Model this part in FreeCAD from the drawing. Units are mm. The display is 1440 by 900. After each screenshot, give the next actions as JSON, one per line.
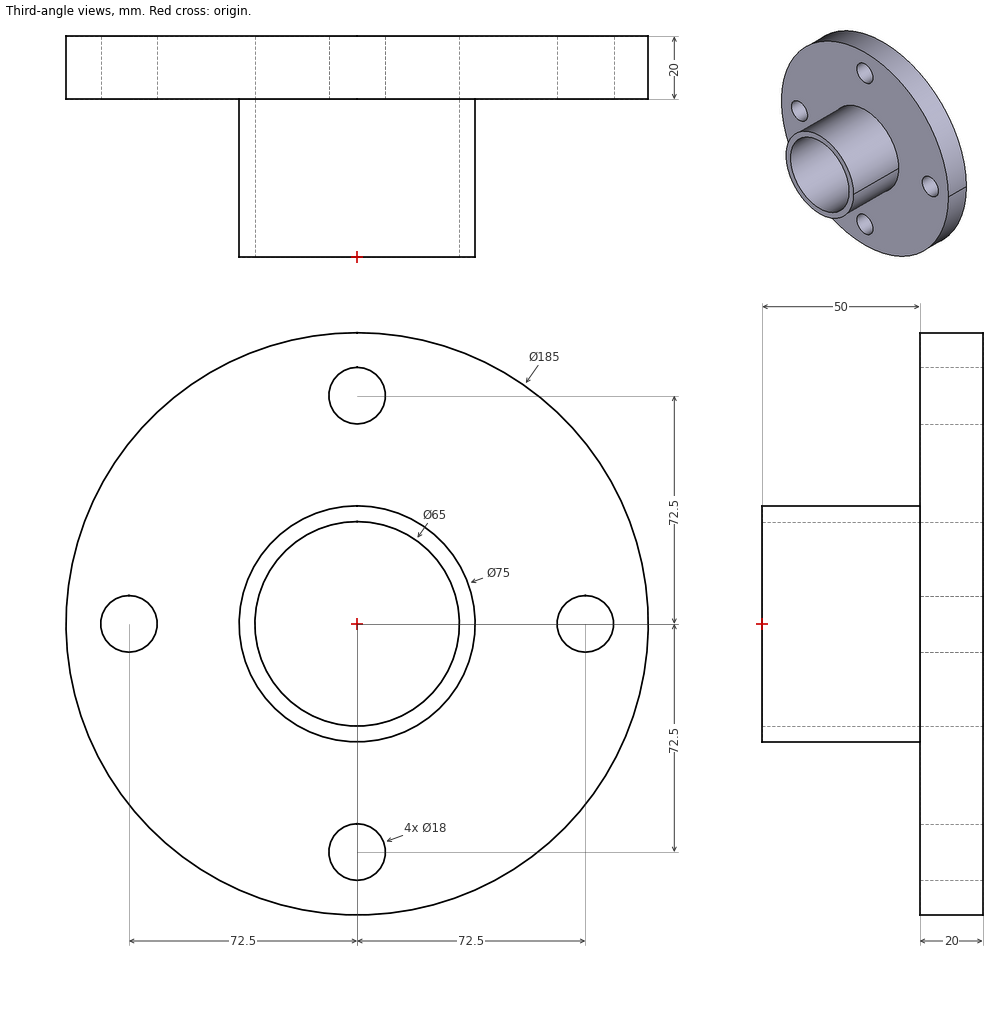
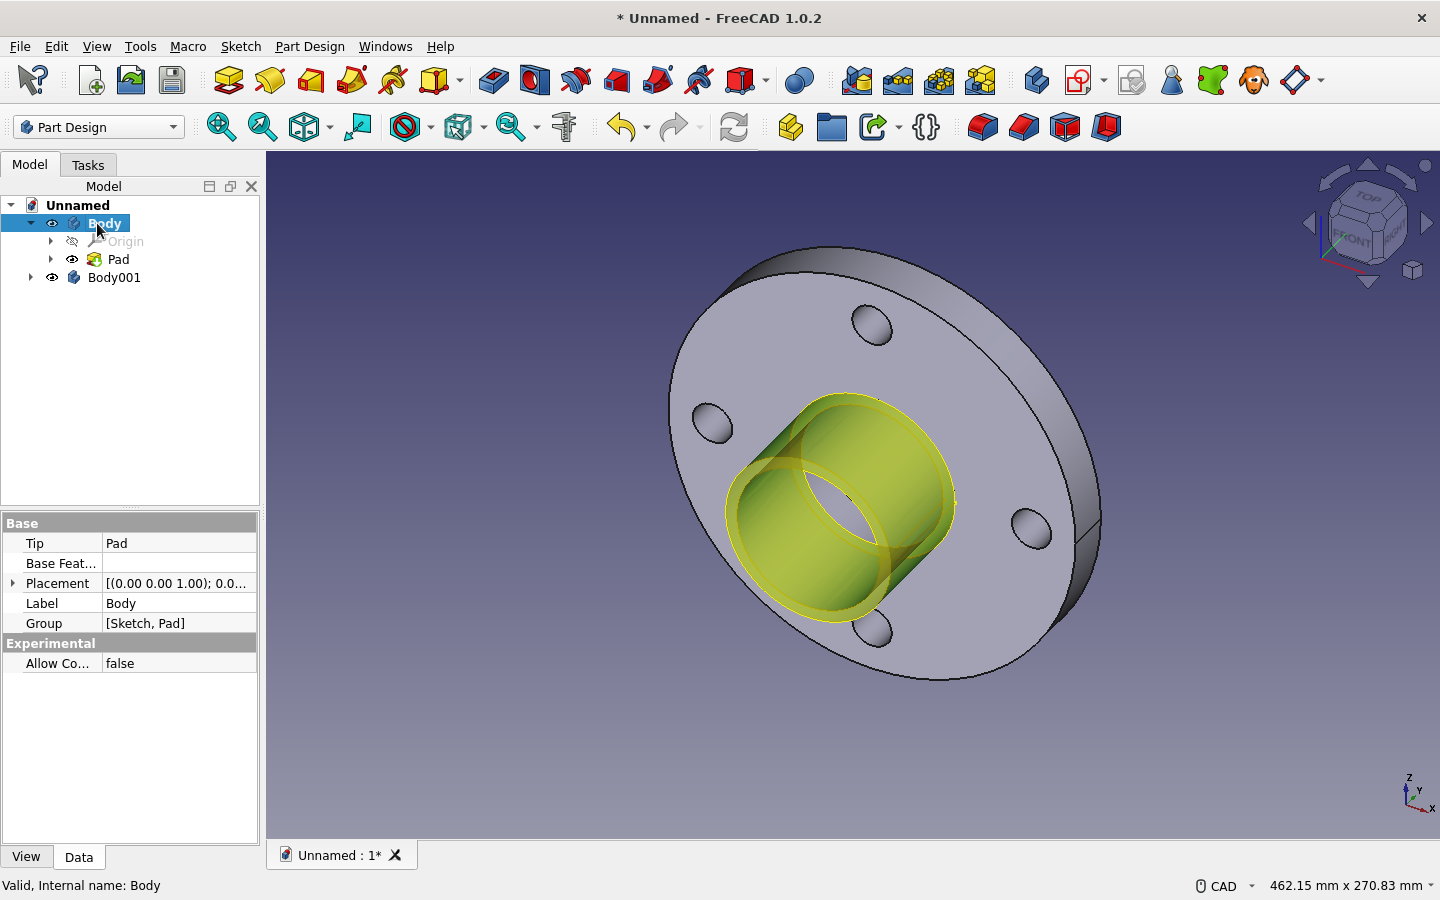
{"action": "left_click", "coordinate": [148, 663]}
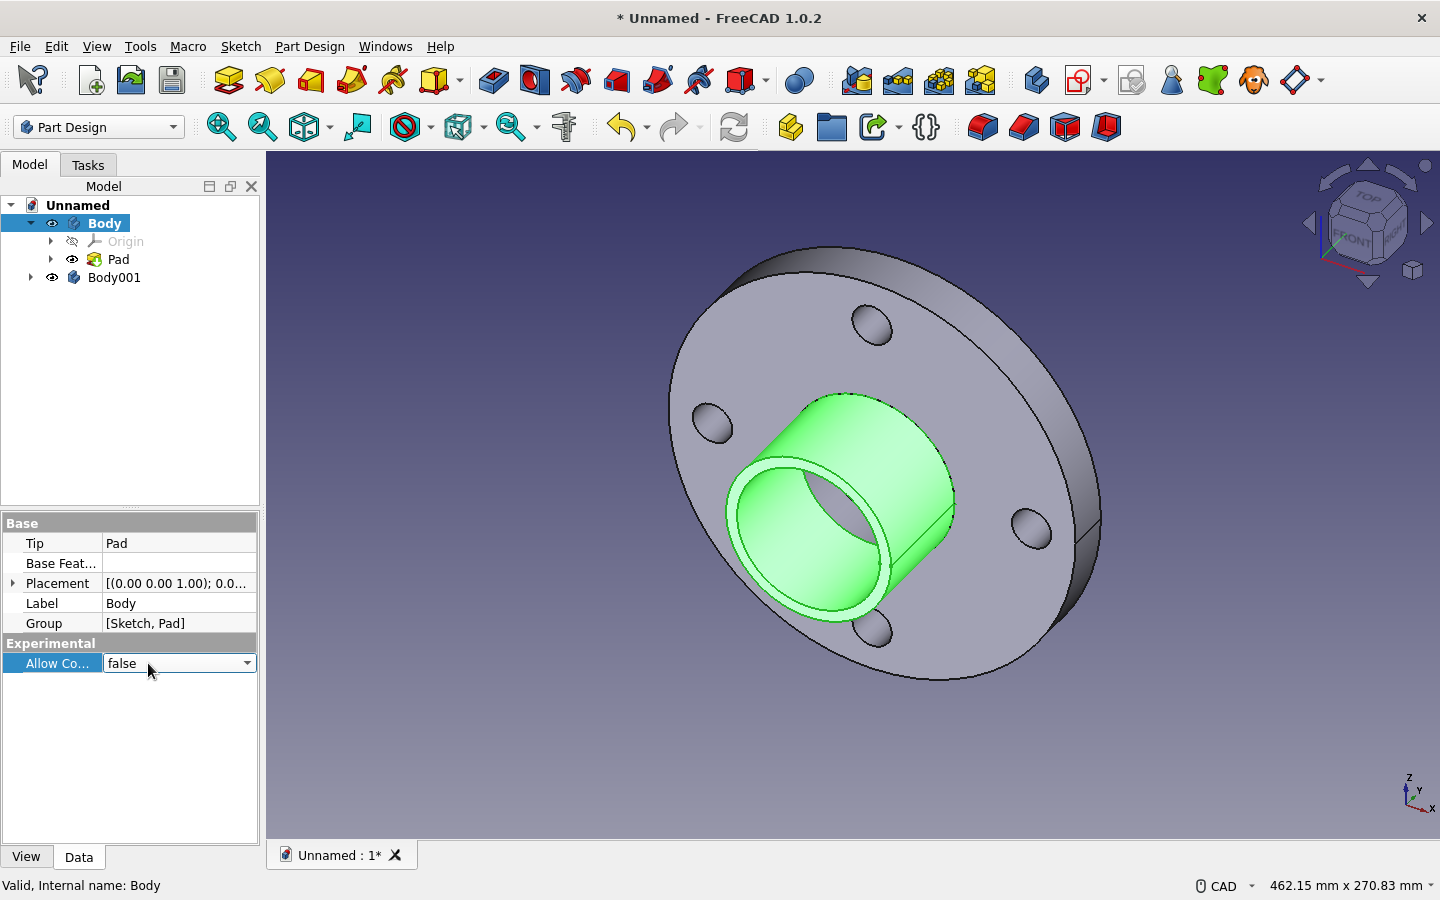
{"action": "left_click", "coordinate": [148, 663]}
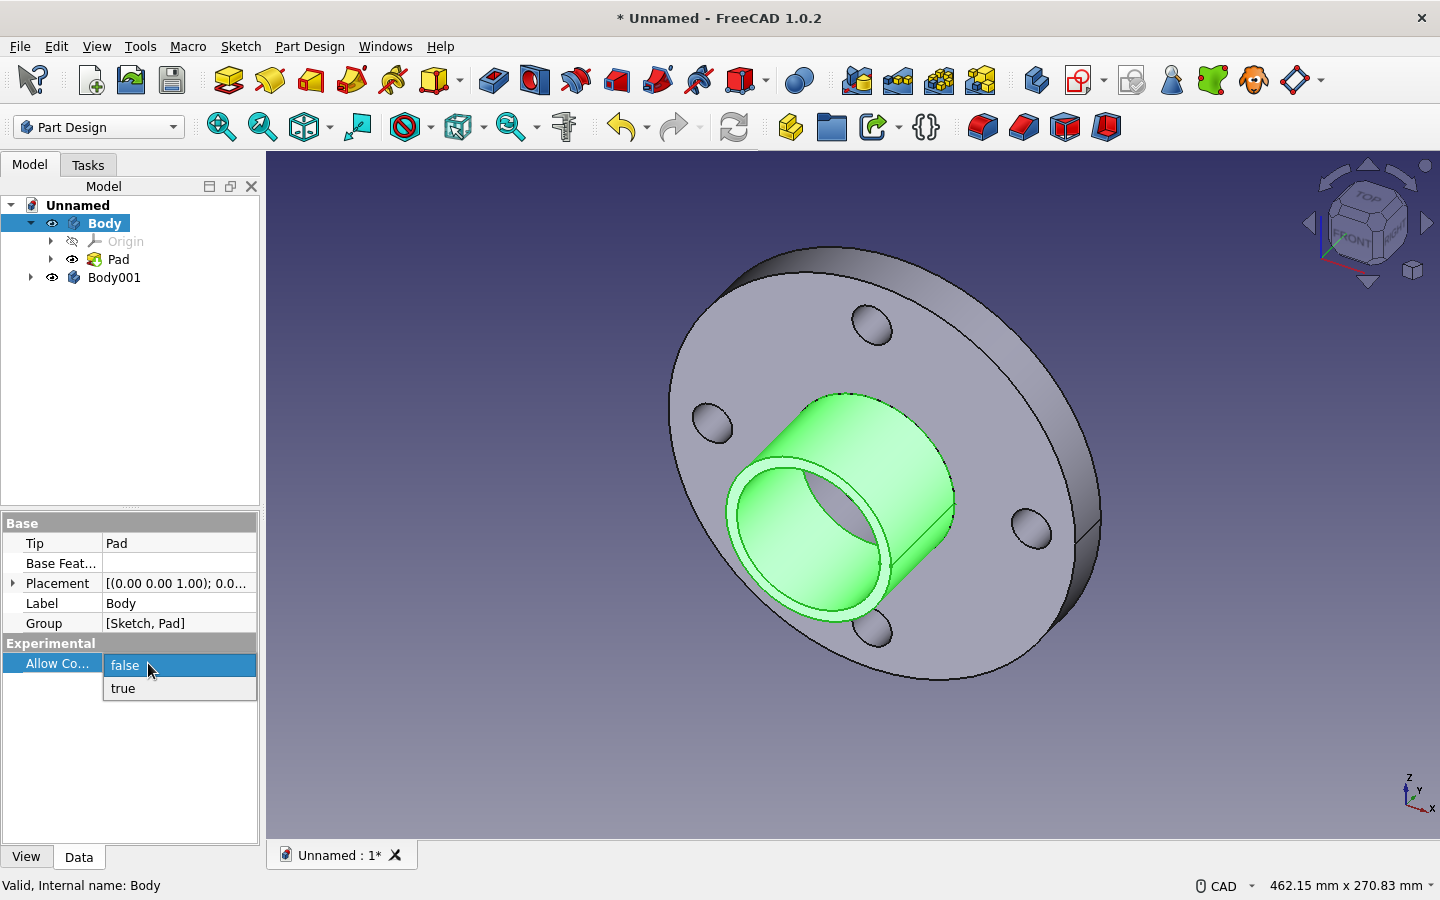
{"action": "left_click", "coordinate": [178, 688]}
{"action": "key", "text": "Return"}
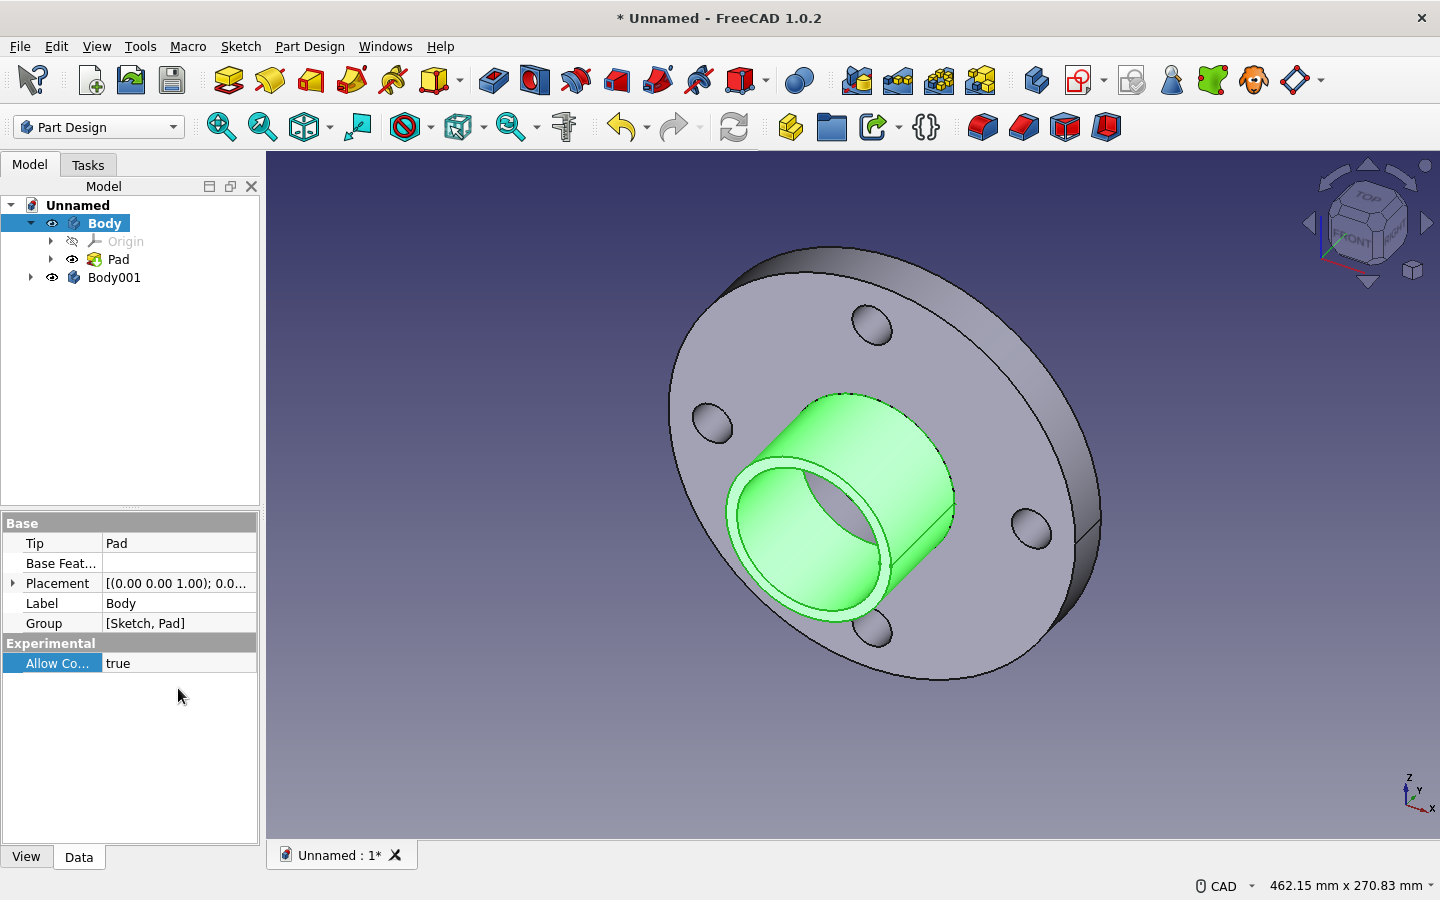
{"action": "left_click", "coordinate": [97, 277]}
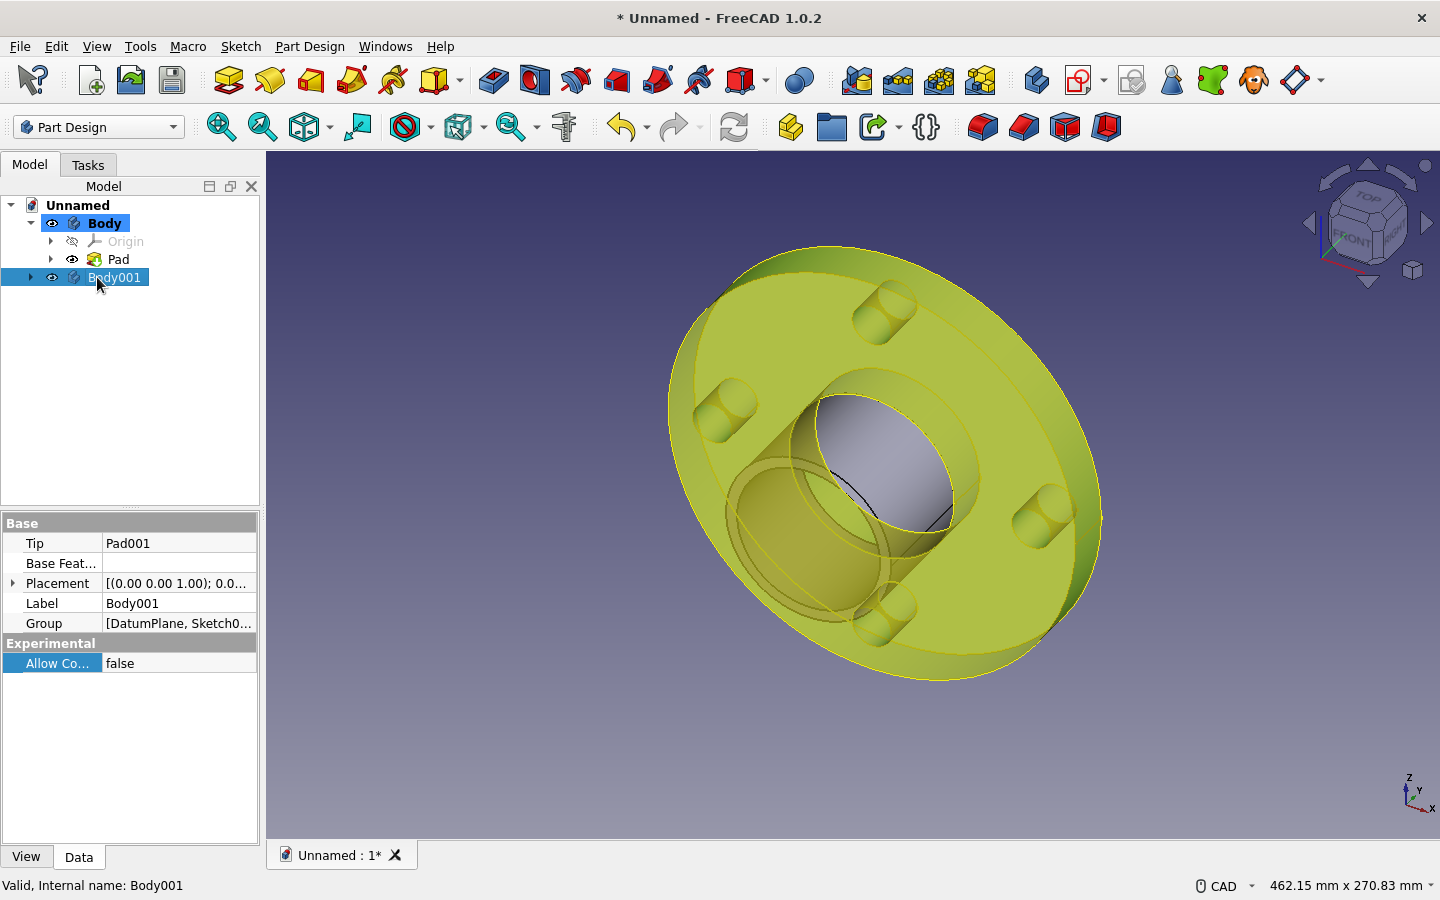
{"action": "left_click", "coordinate": [800, 80]}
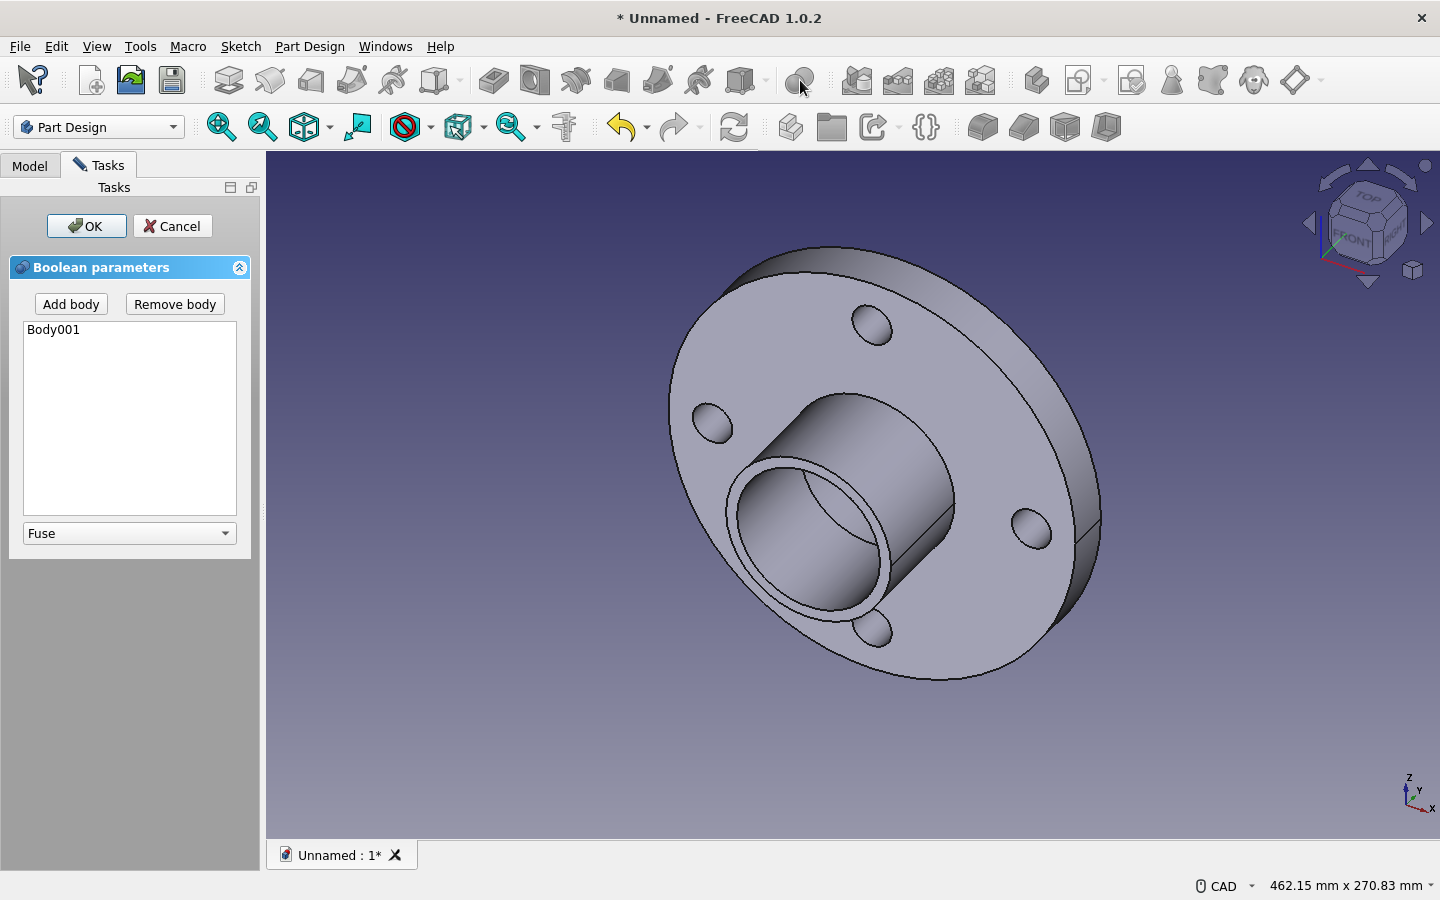
{"action": "left_click", "coordinate": [87, 226]}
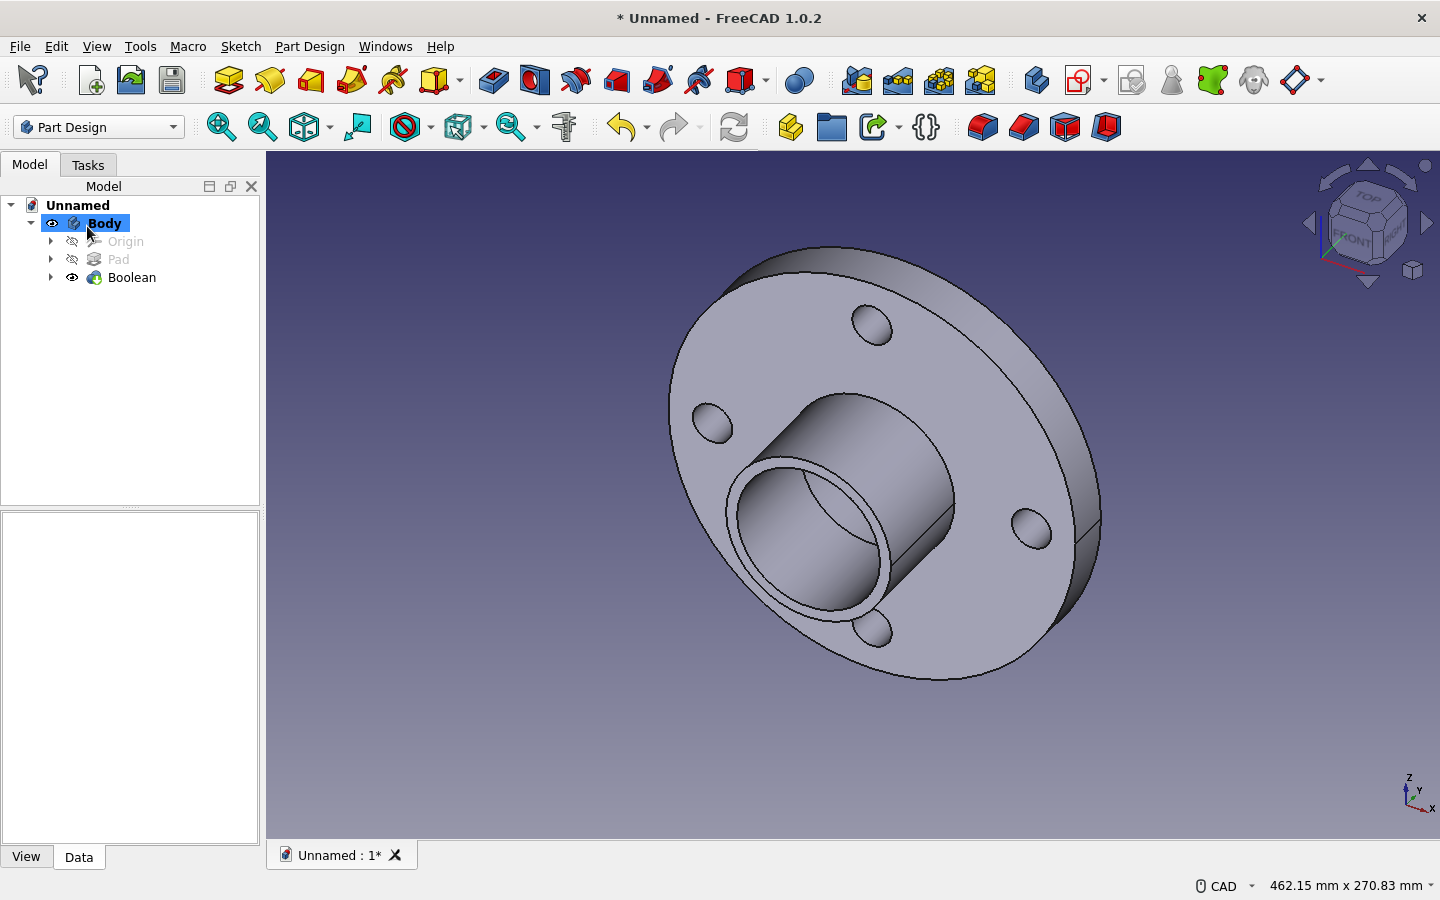
{"action": "left_click", "coordinate": [814, 346]}